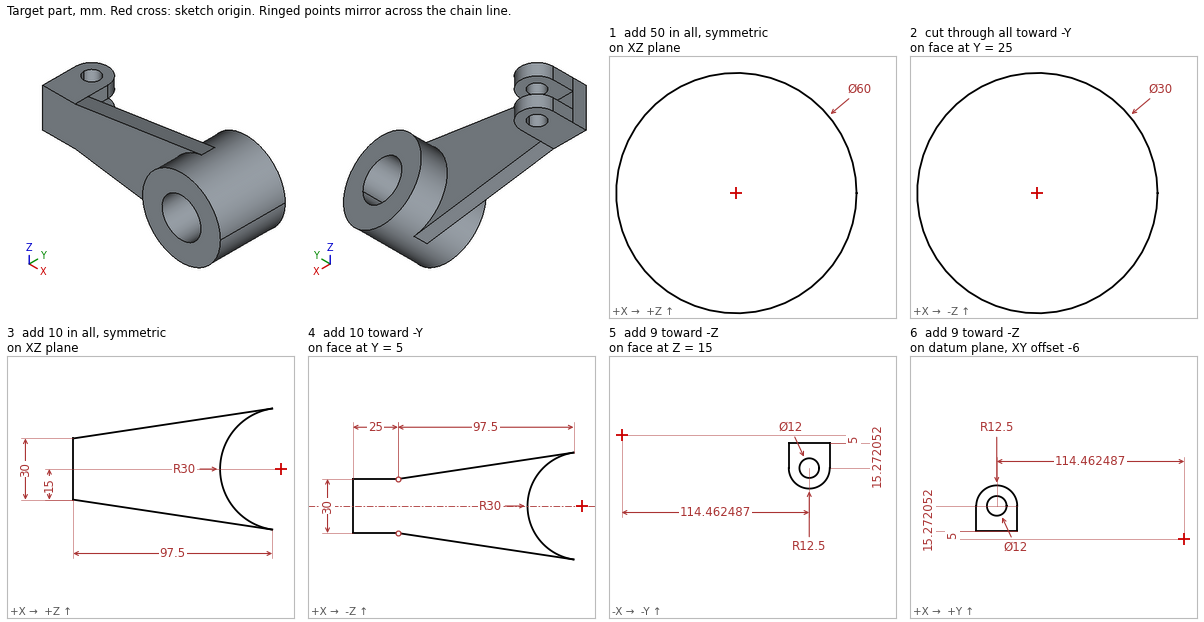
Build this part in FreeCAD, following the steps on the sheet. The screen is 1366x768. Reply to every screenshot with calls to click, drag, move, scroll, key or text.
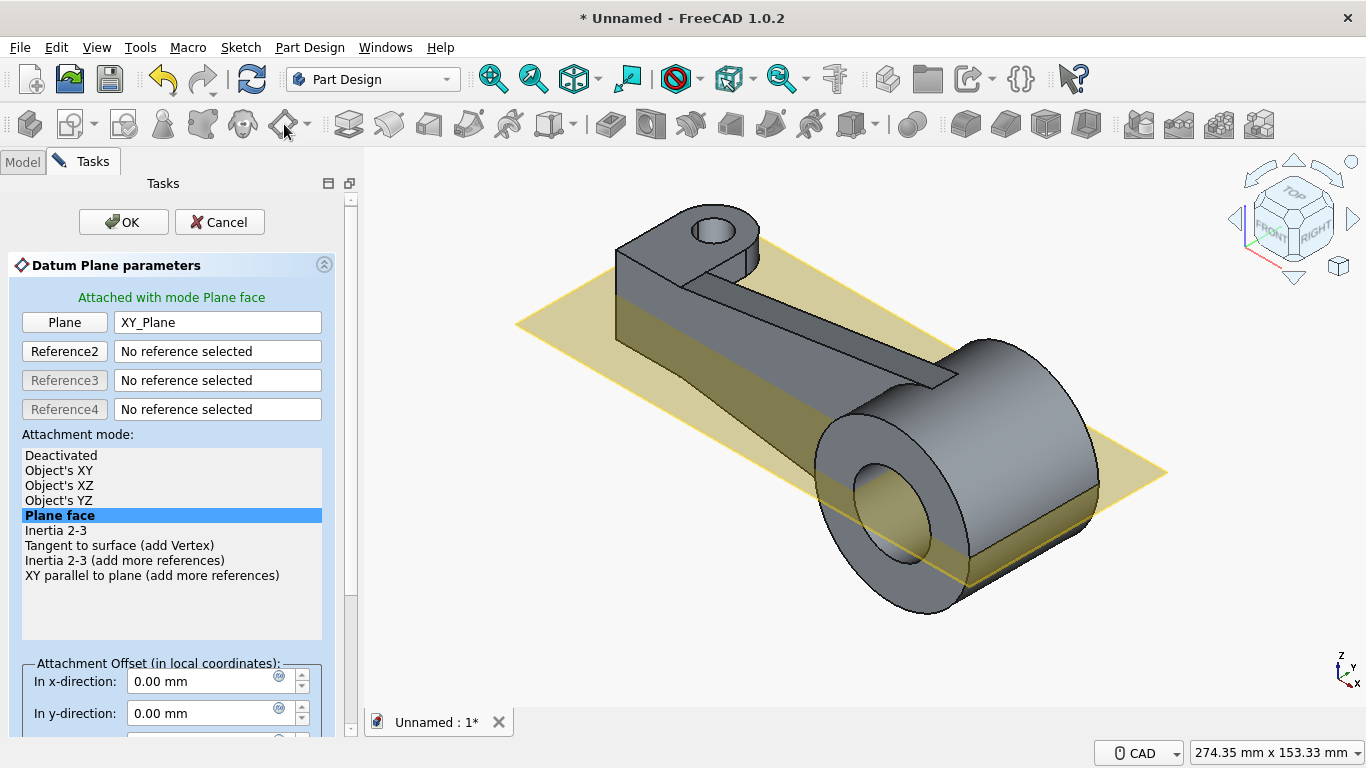
scroll(351, 464, down, 2)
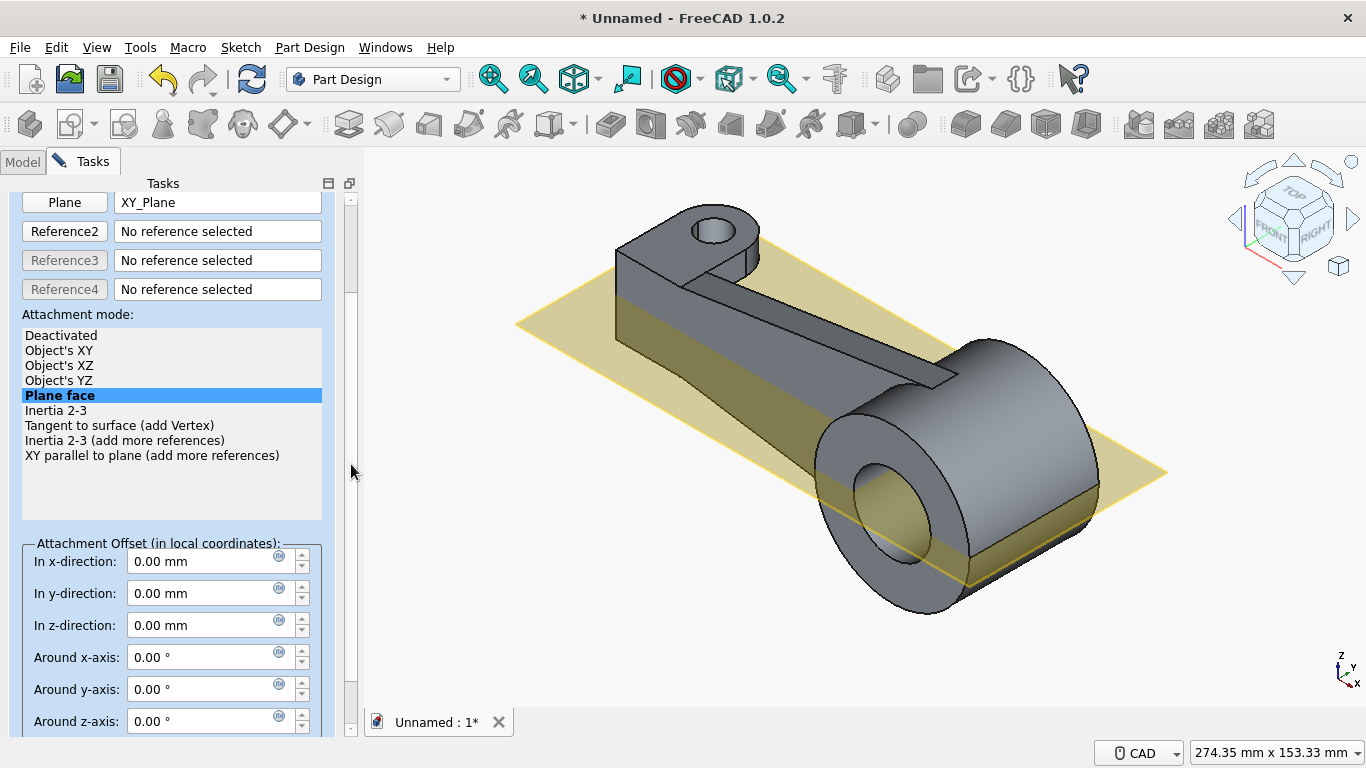
triple_click(210, 625)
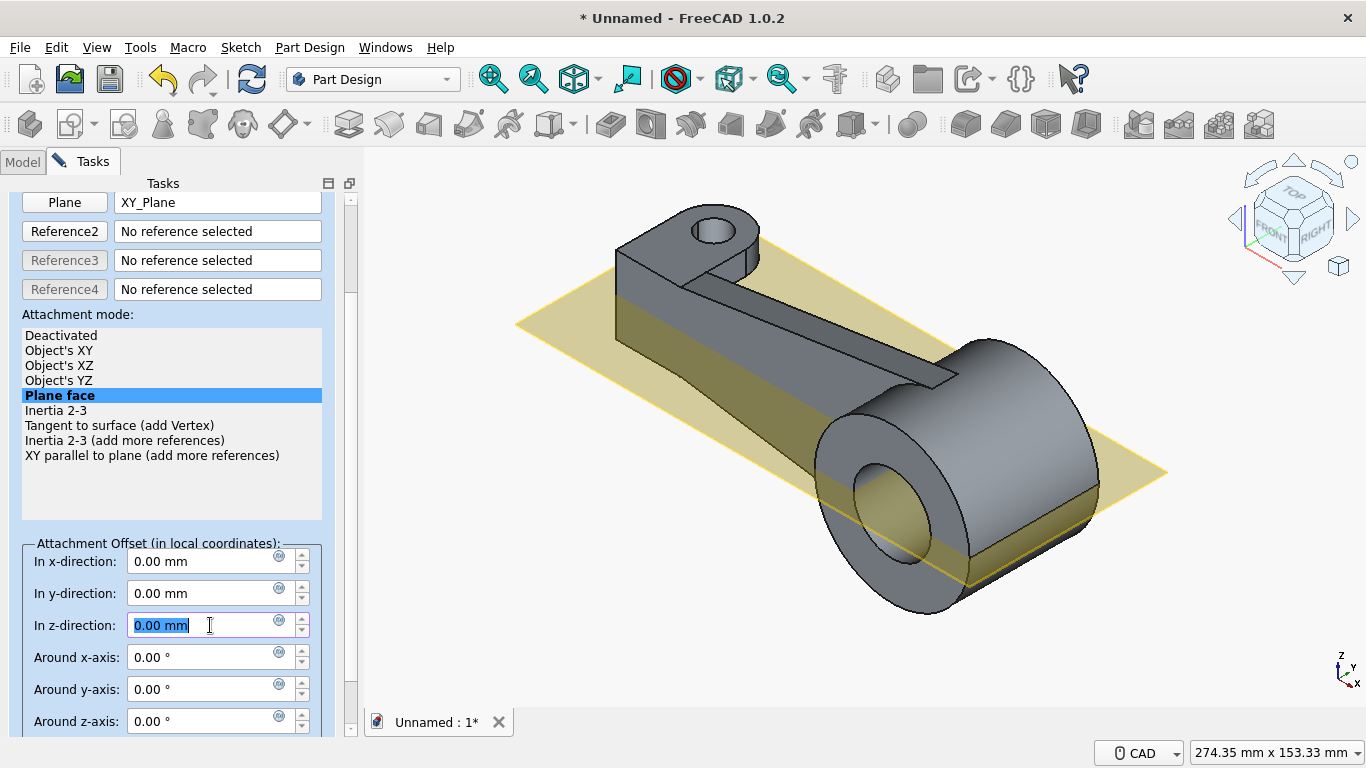
text(-6)
key(Tab)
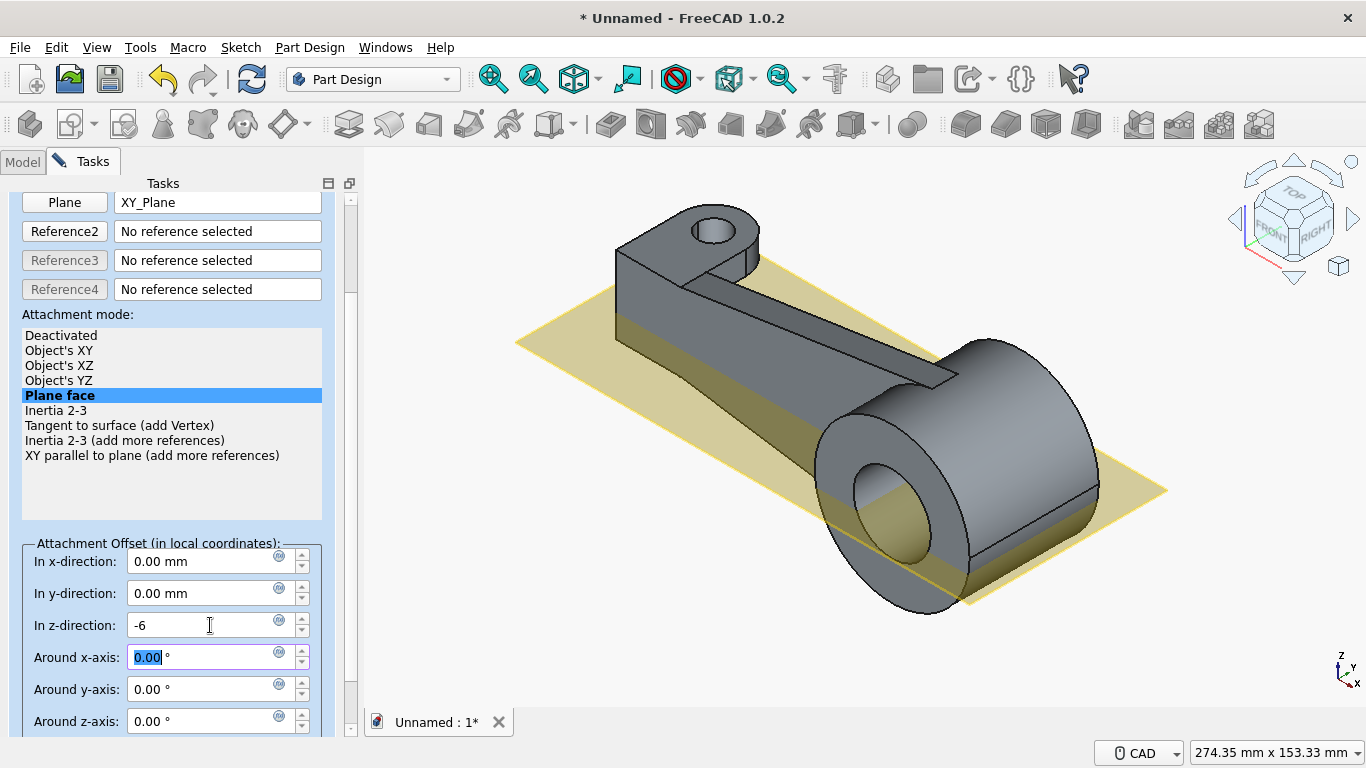
scroll(351, 464, up, 3)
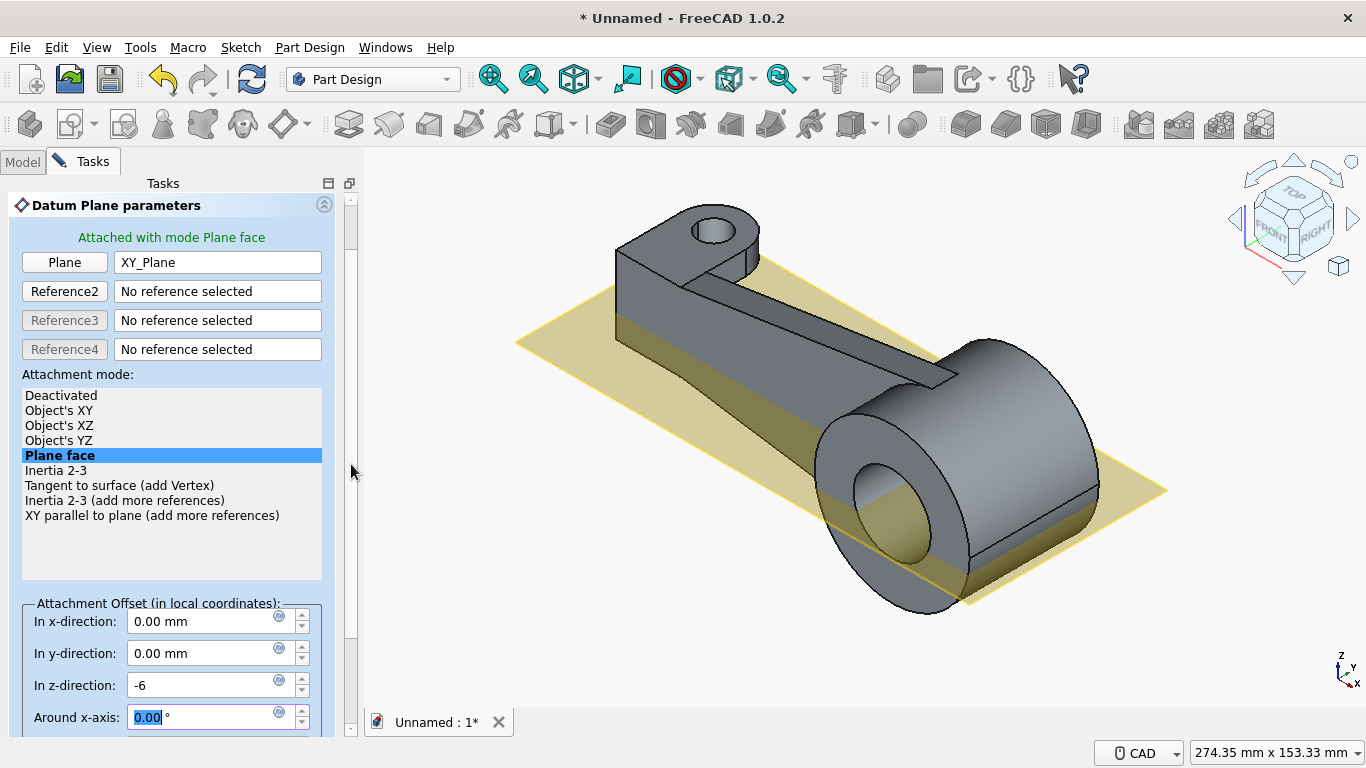
click(124, 222)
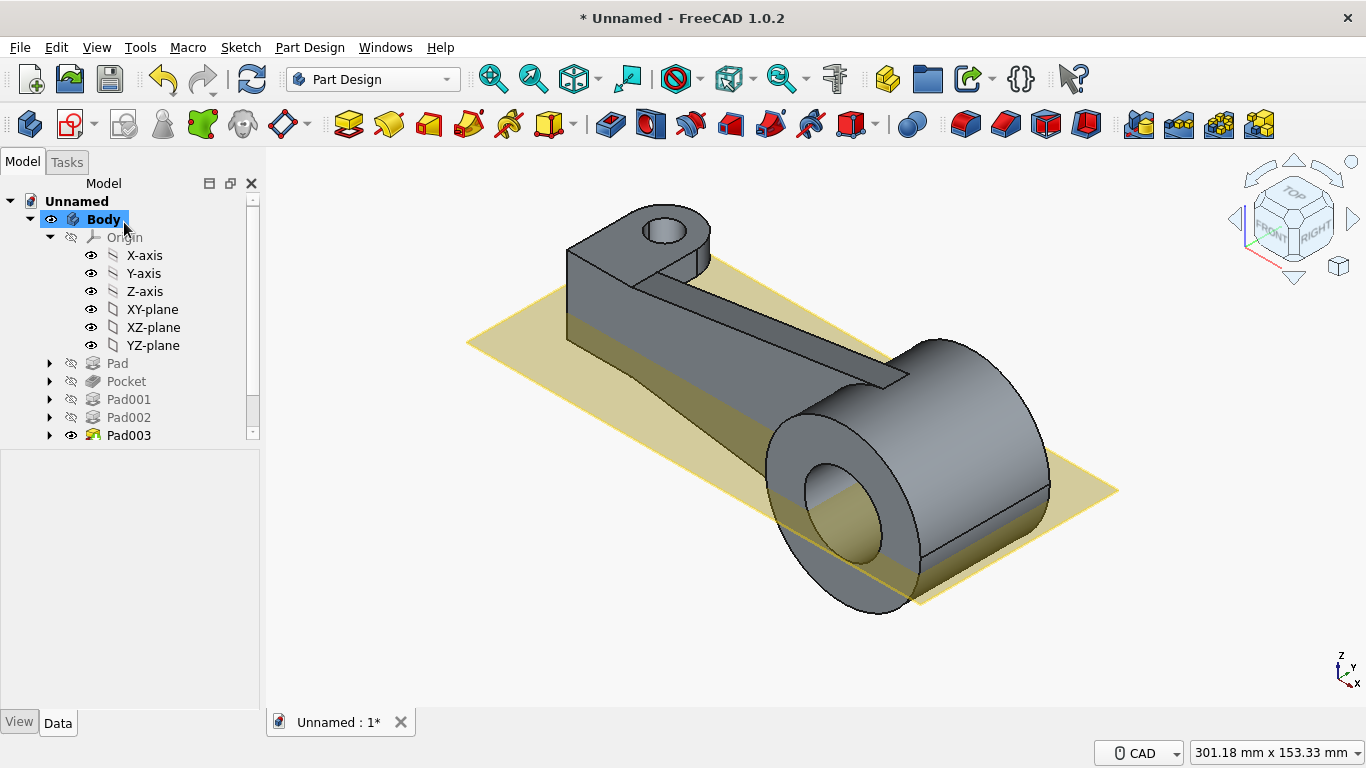
scroll(100, 323, down, 3)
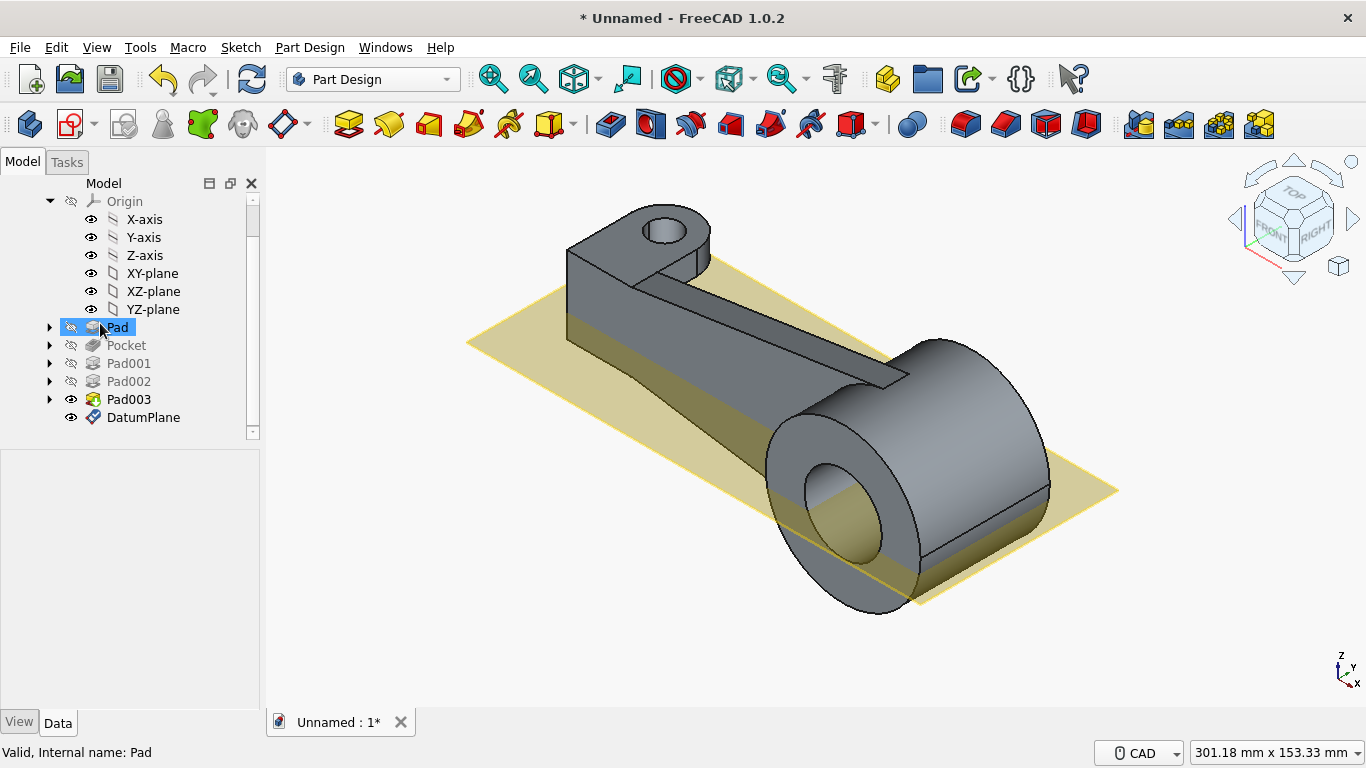
click(116, 417)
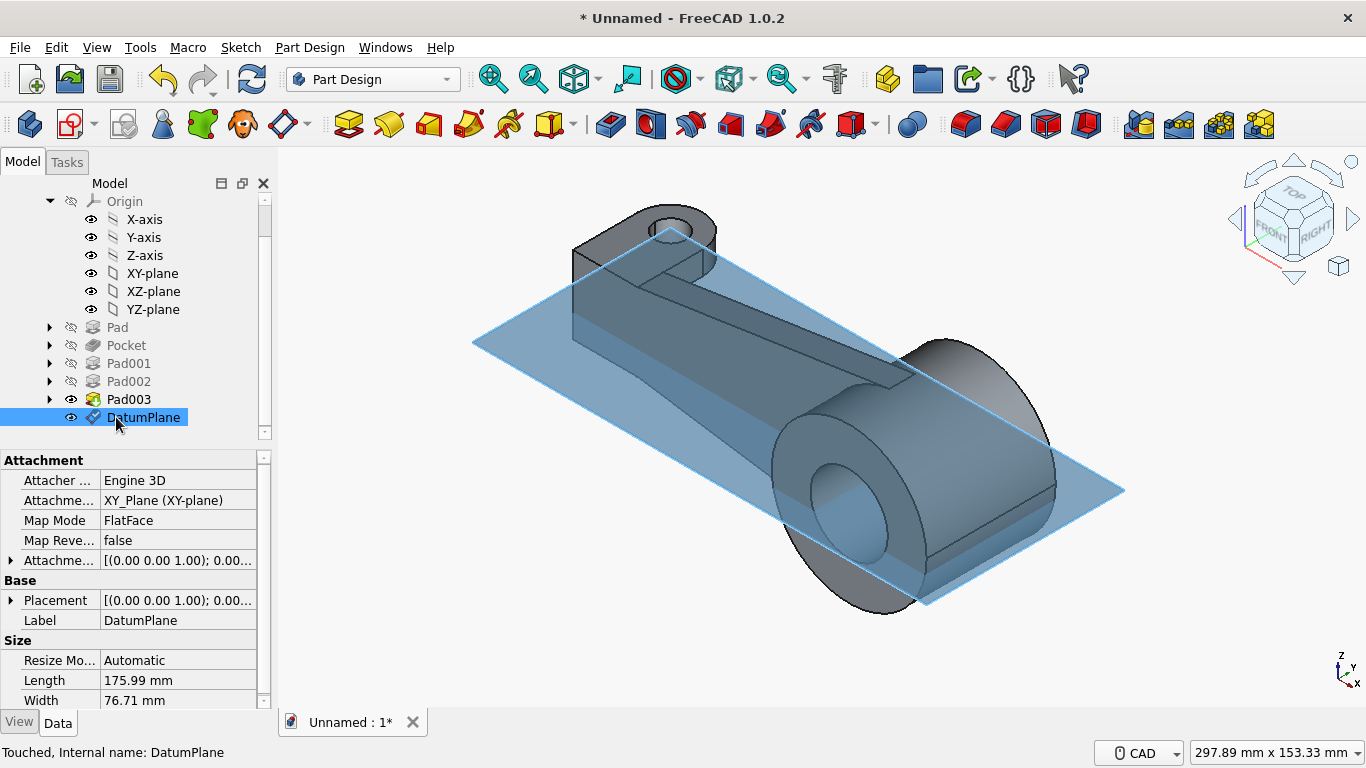
click(70, 124)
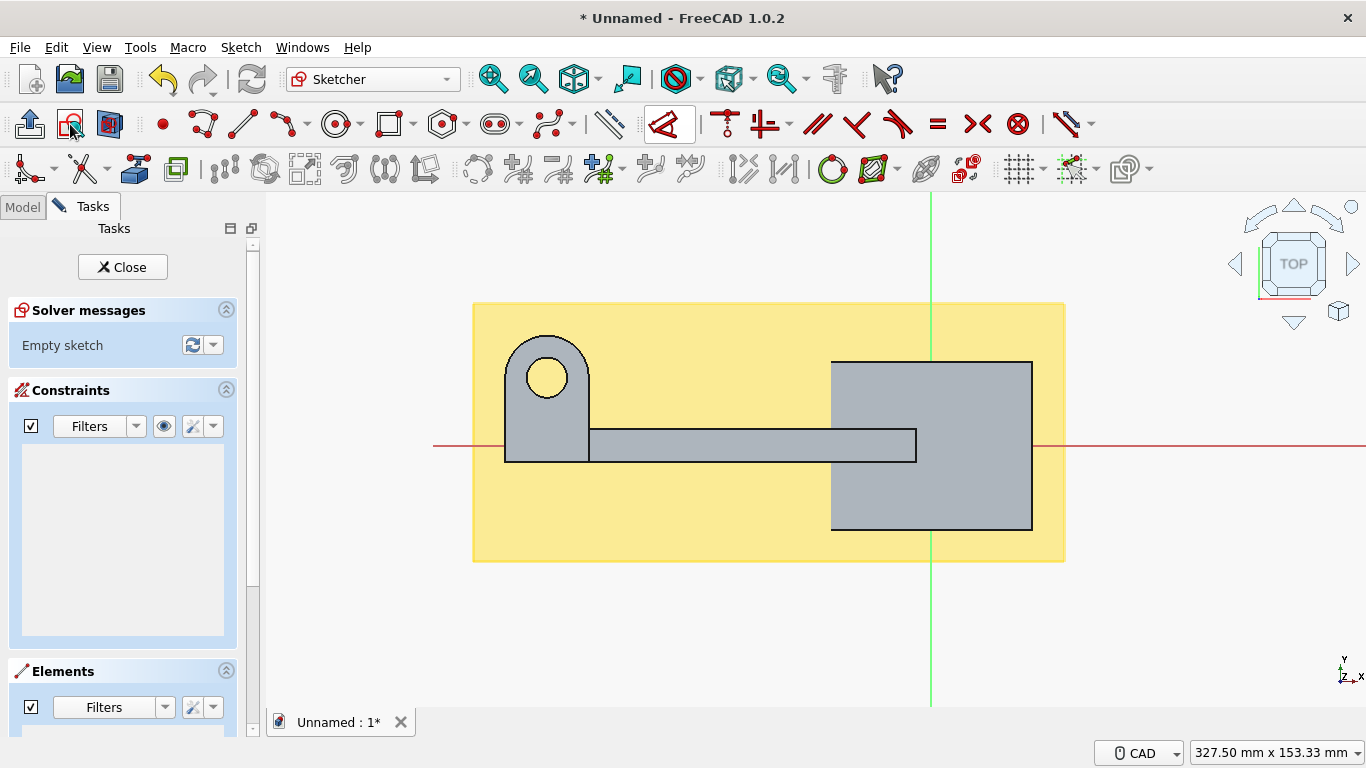
click(110, 124)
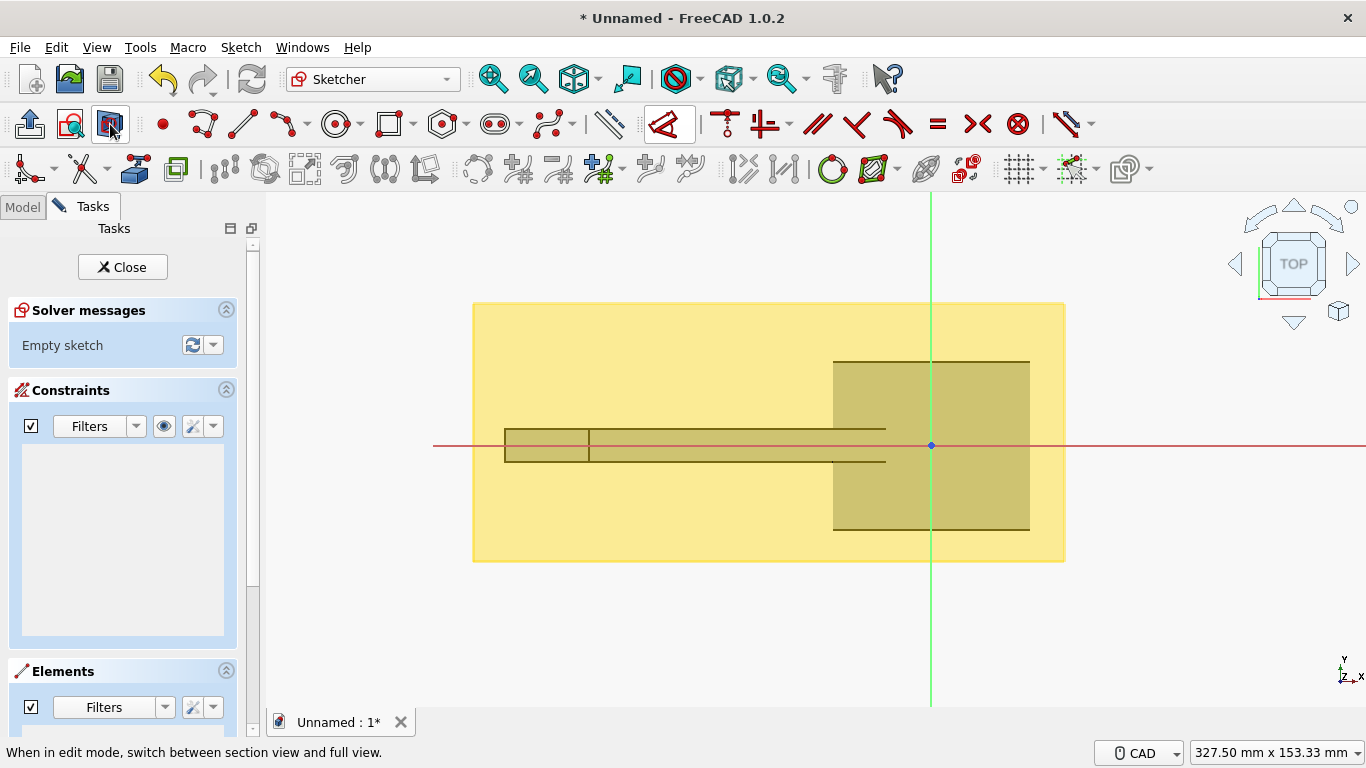
scroll(461, 353, up, 6)